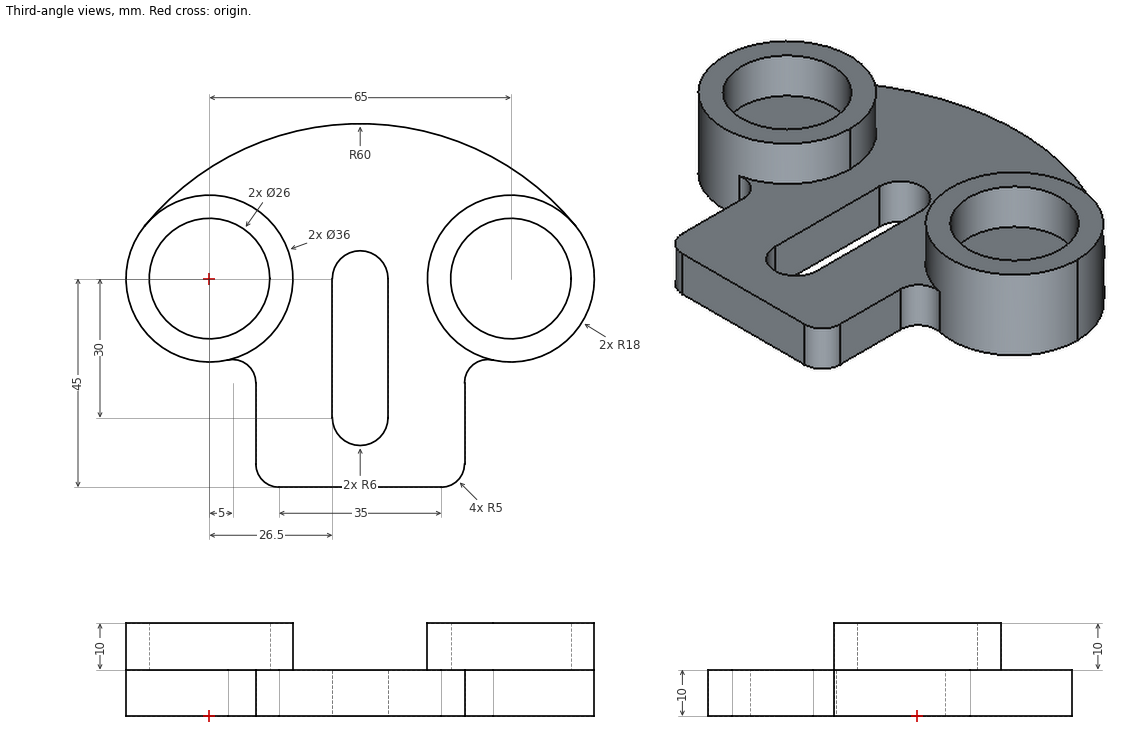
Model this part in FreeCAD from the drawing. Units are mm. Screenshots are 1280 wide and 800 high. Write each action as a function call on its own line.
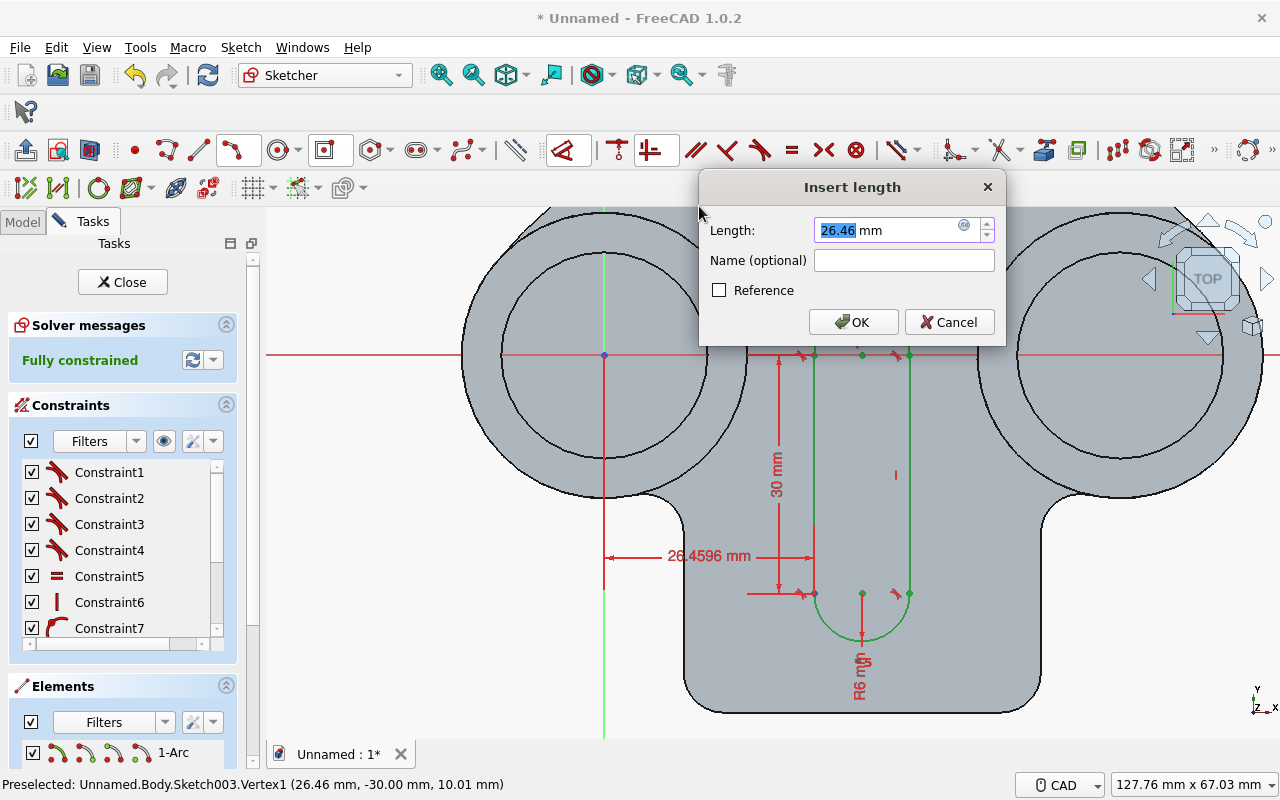
text(26.5)
key(Return)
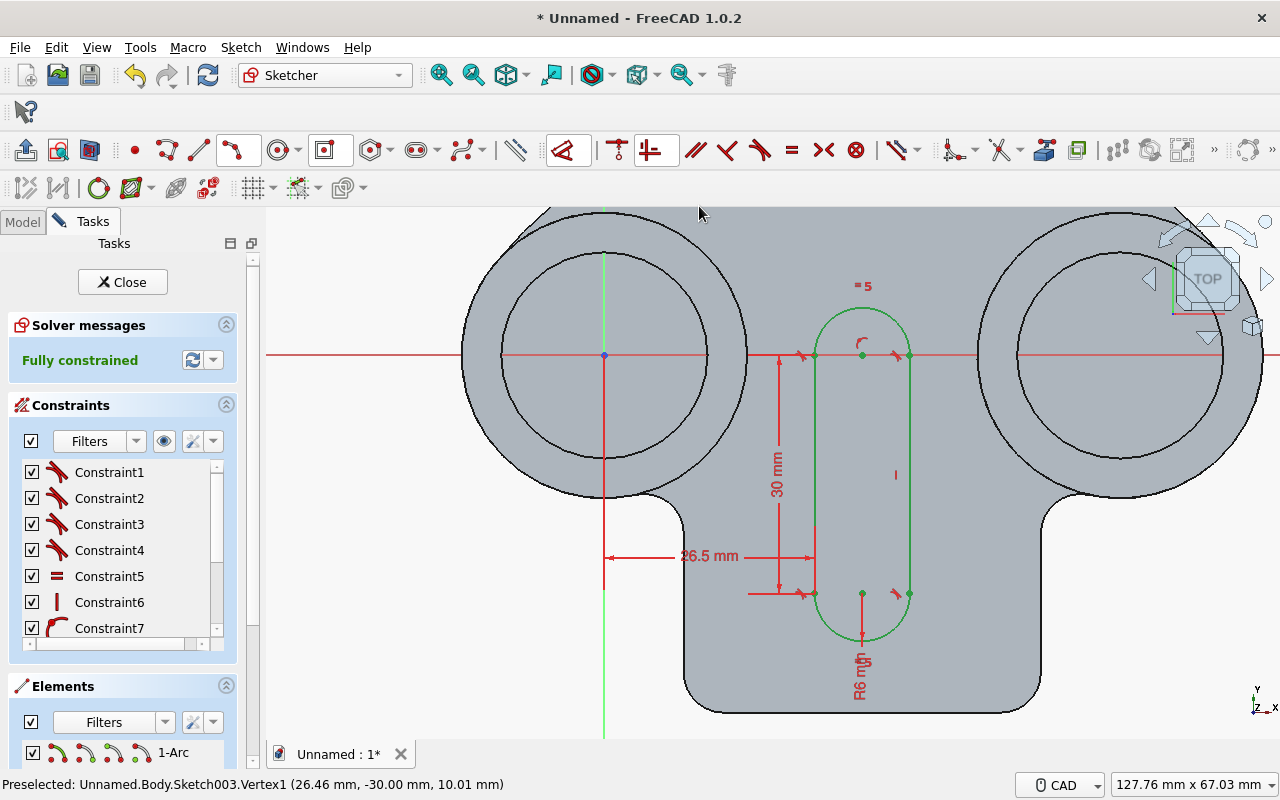
click(123, 282)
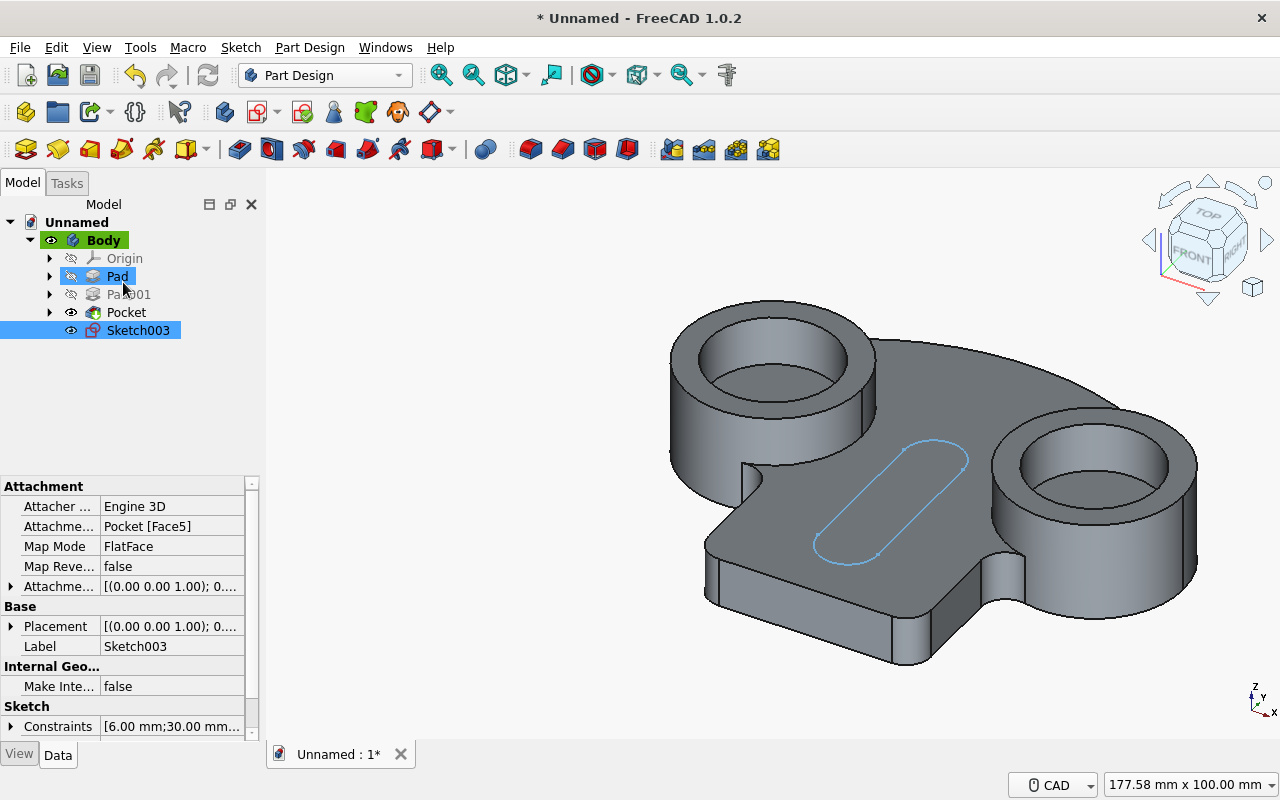
click(240, 150)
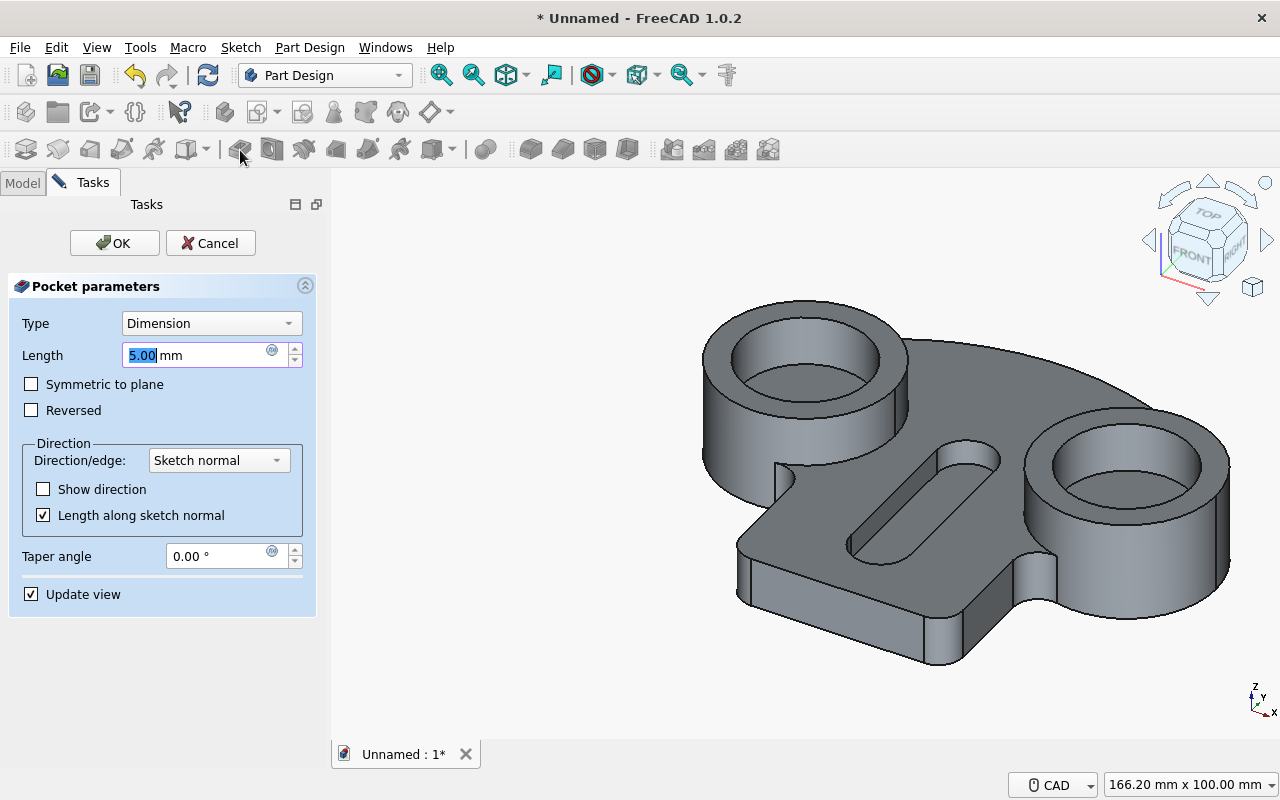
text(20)
key(Tab)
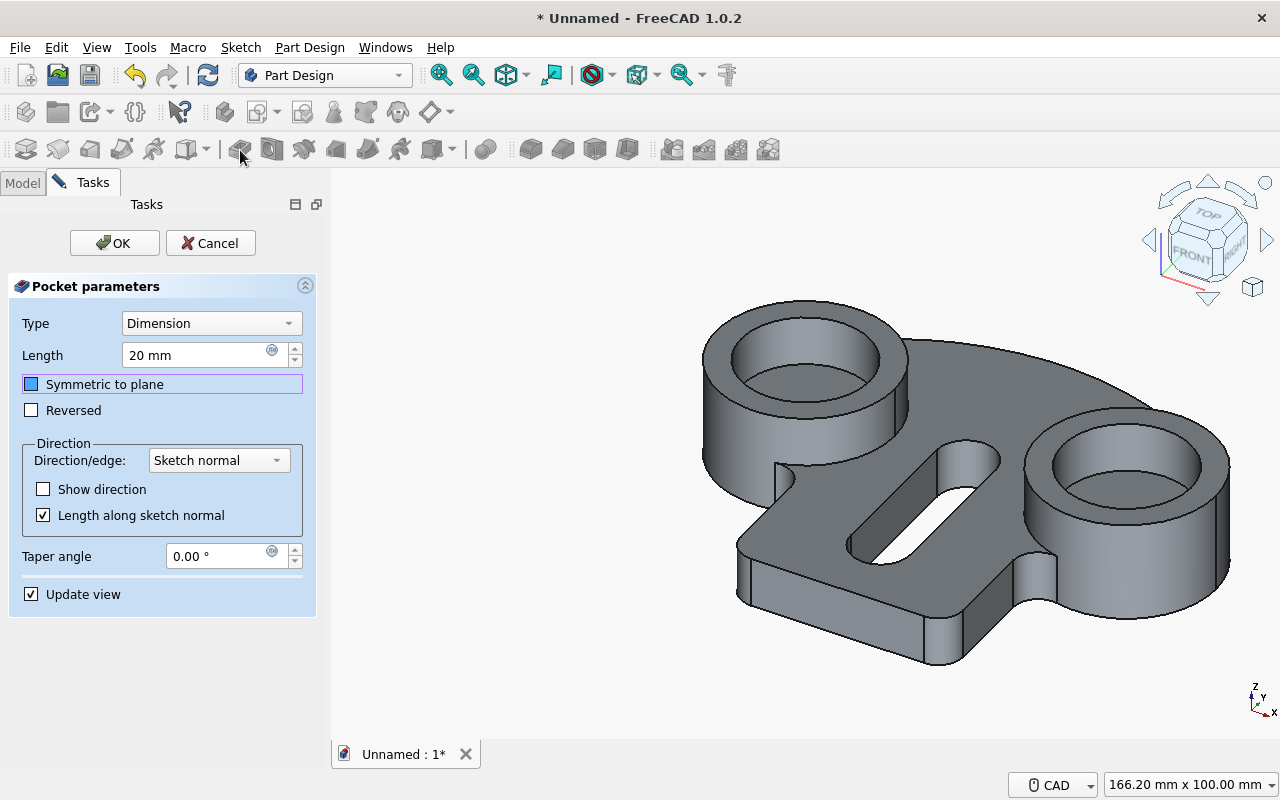
click(115, 243)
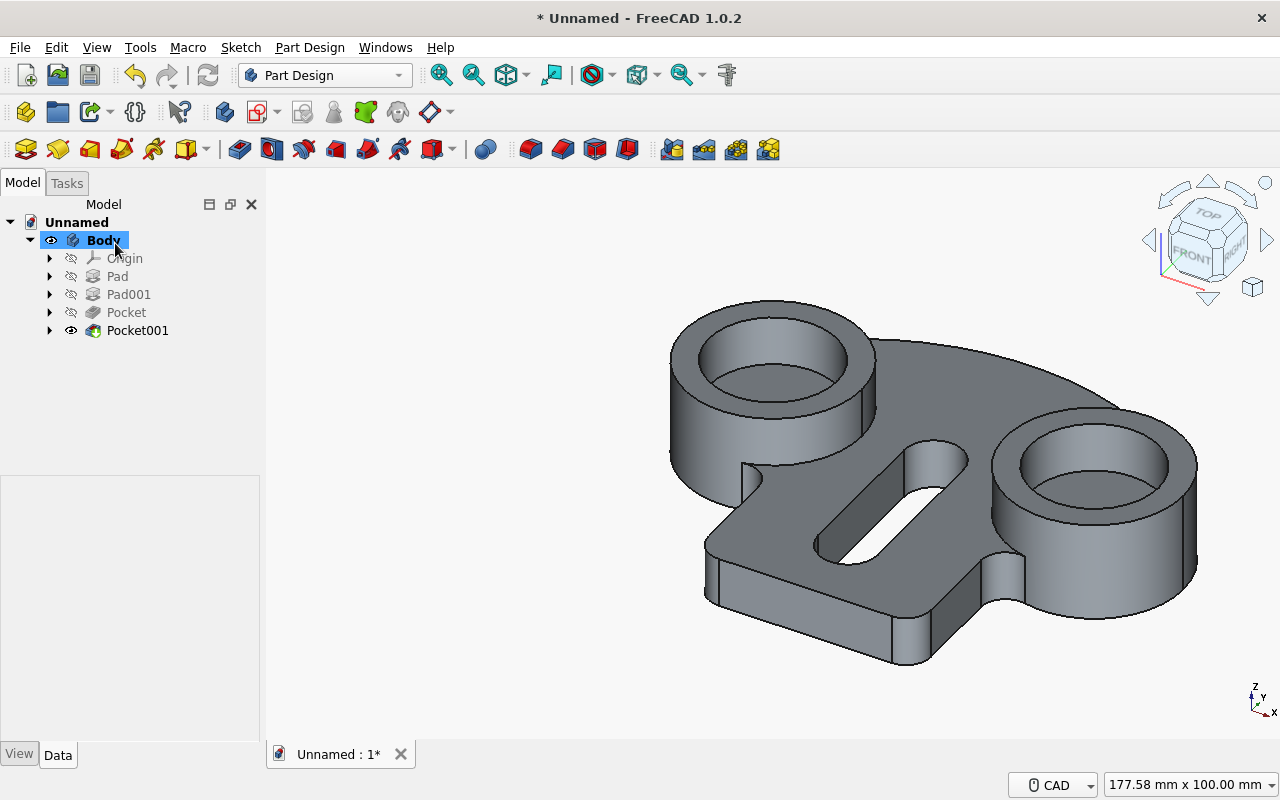
key(0)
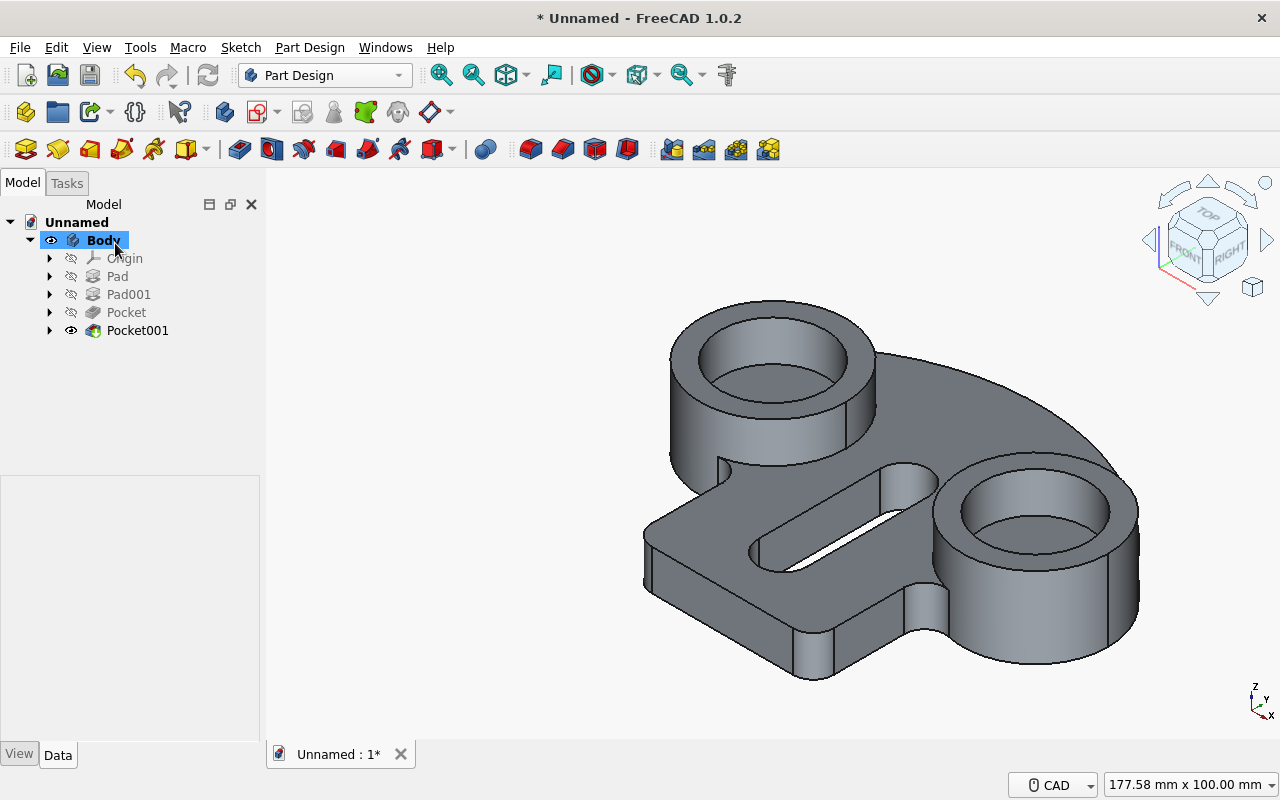
click(442, 76)